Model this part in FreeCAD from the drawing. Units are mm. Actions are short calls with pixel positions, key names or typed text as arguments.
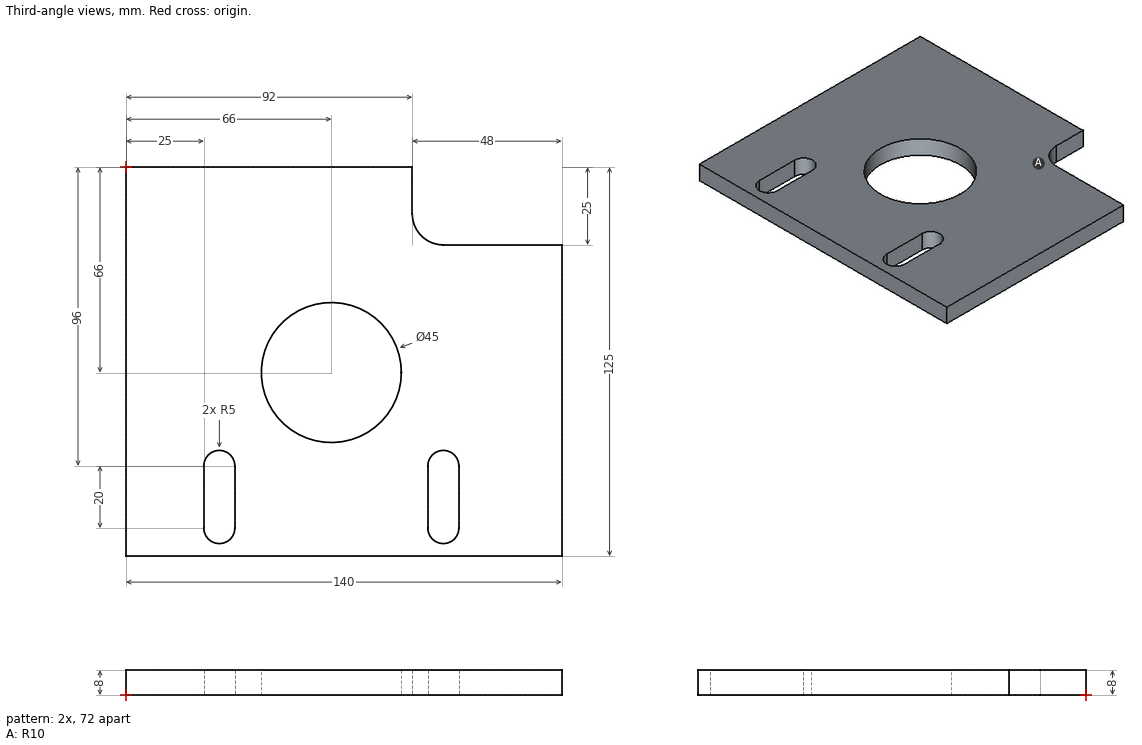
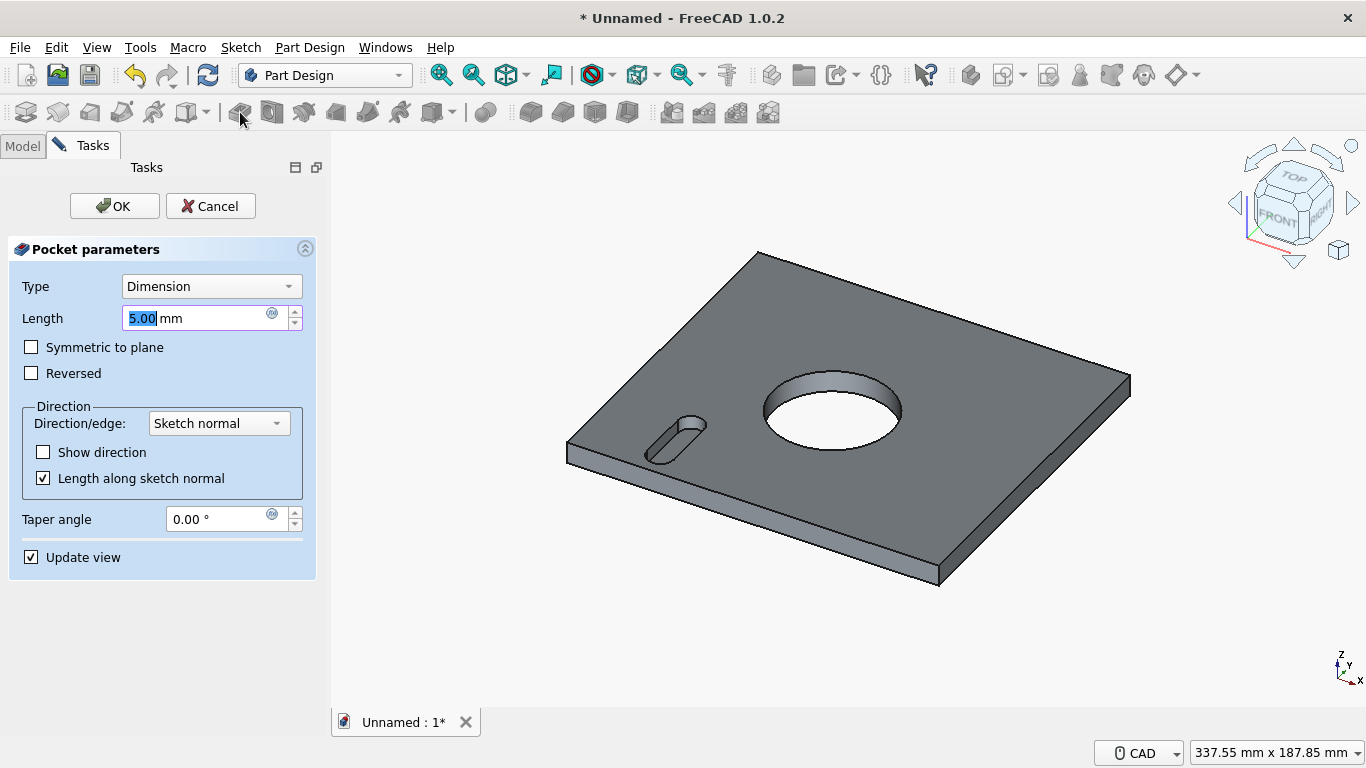
text(8)
key(Tab)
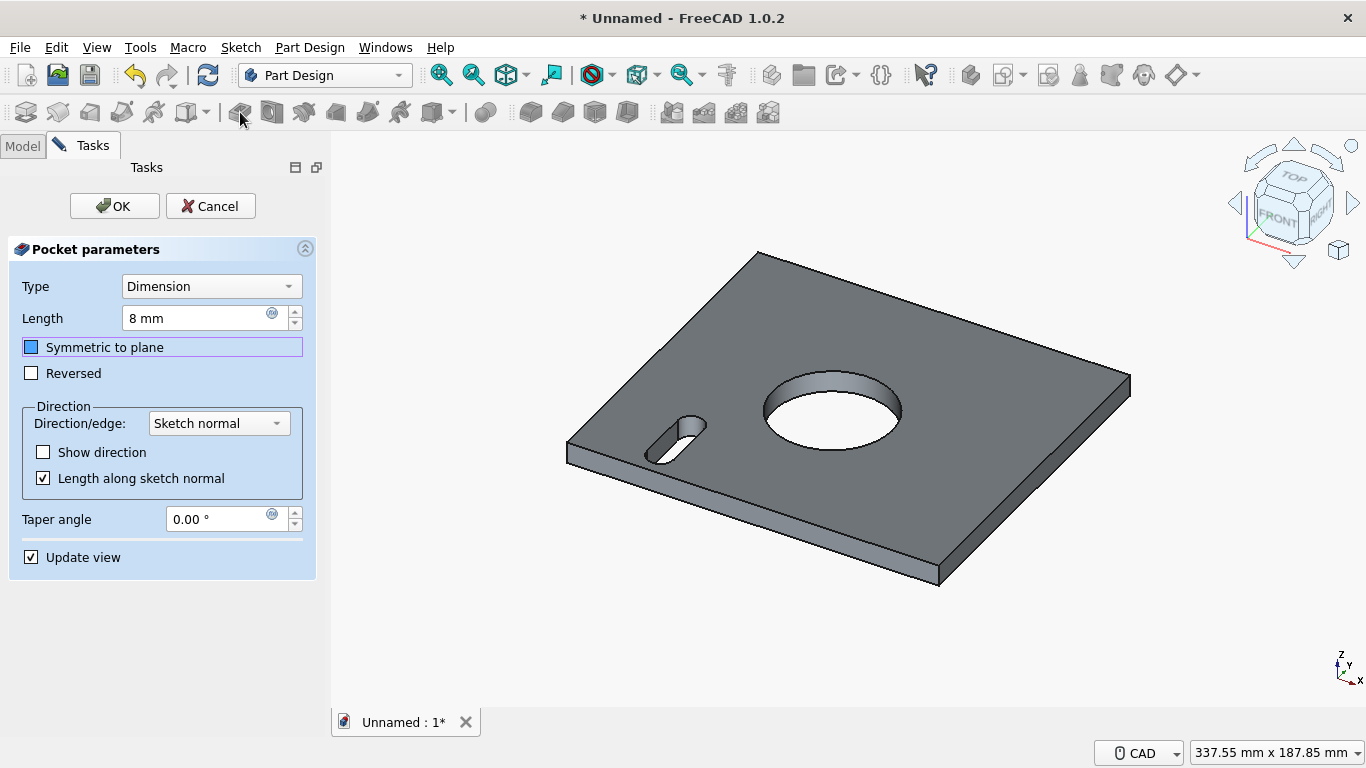
click(115, 206)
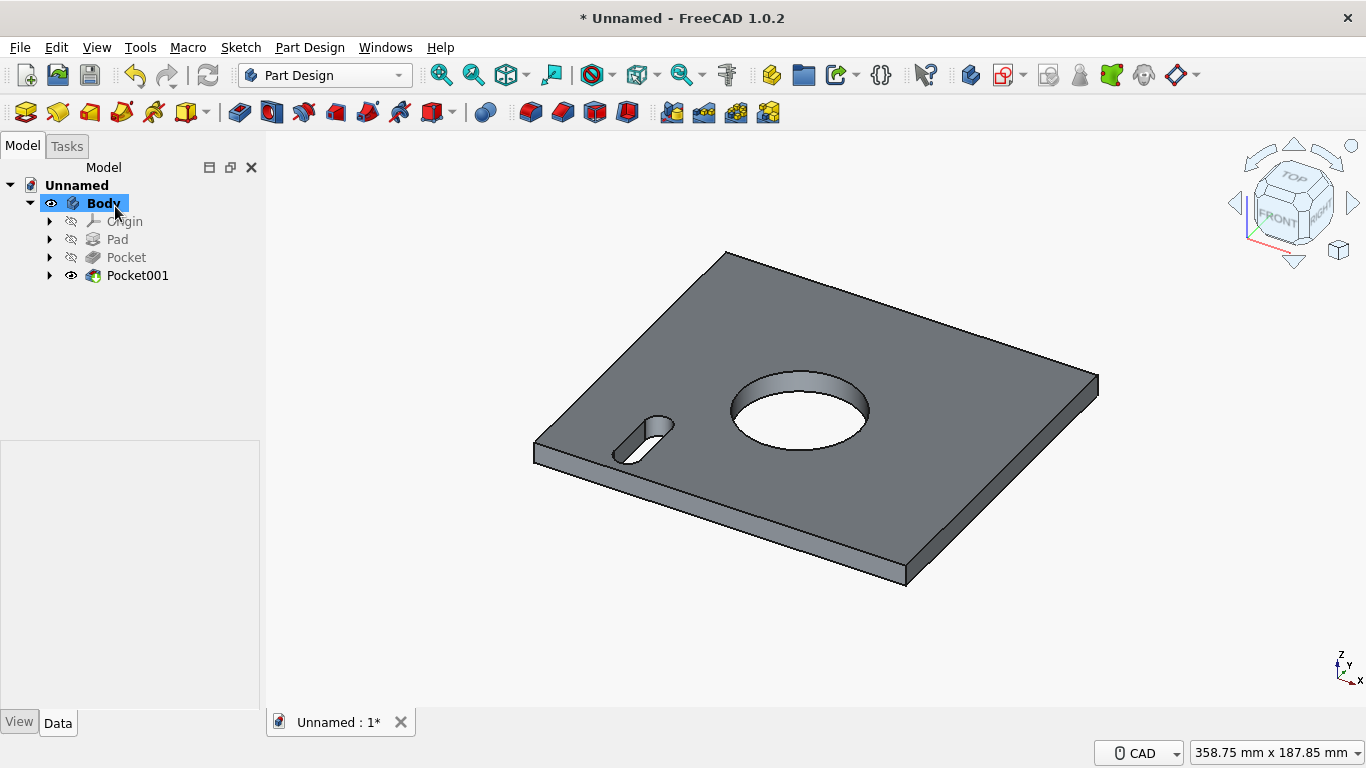
click(116, 275)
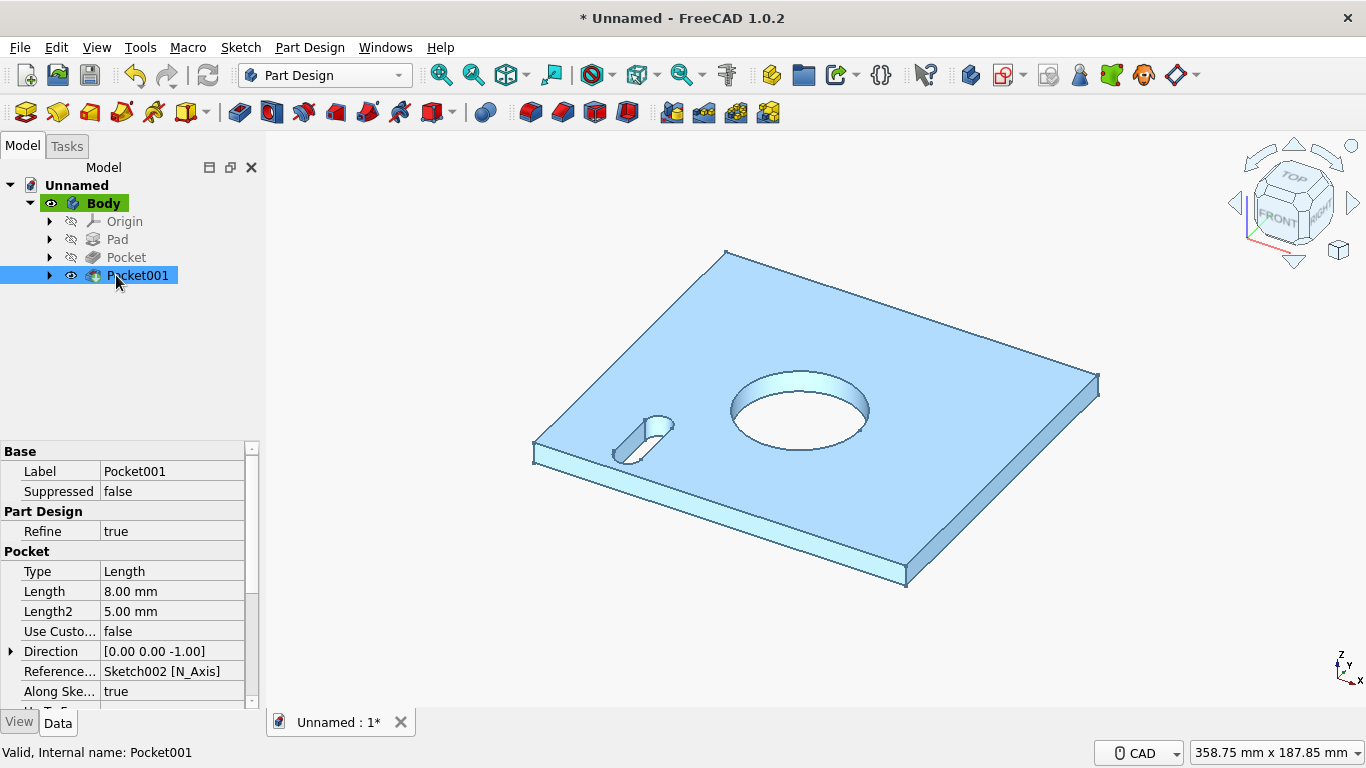
click(704, 112)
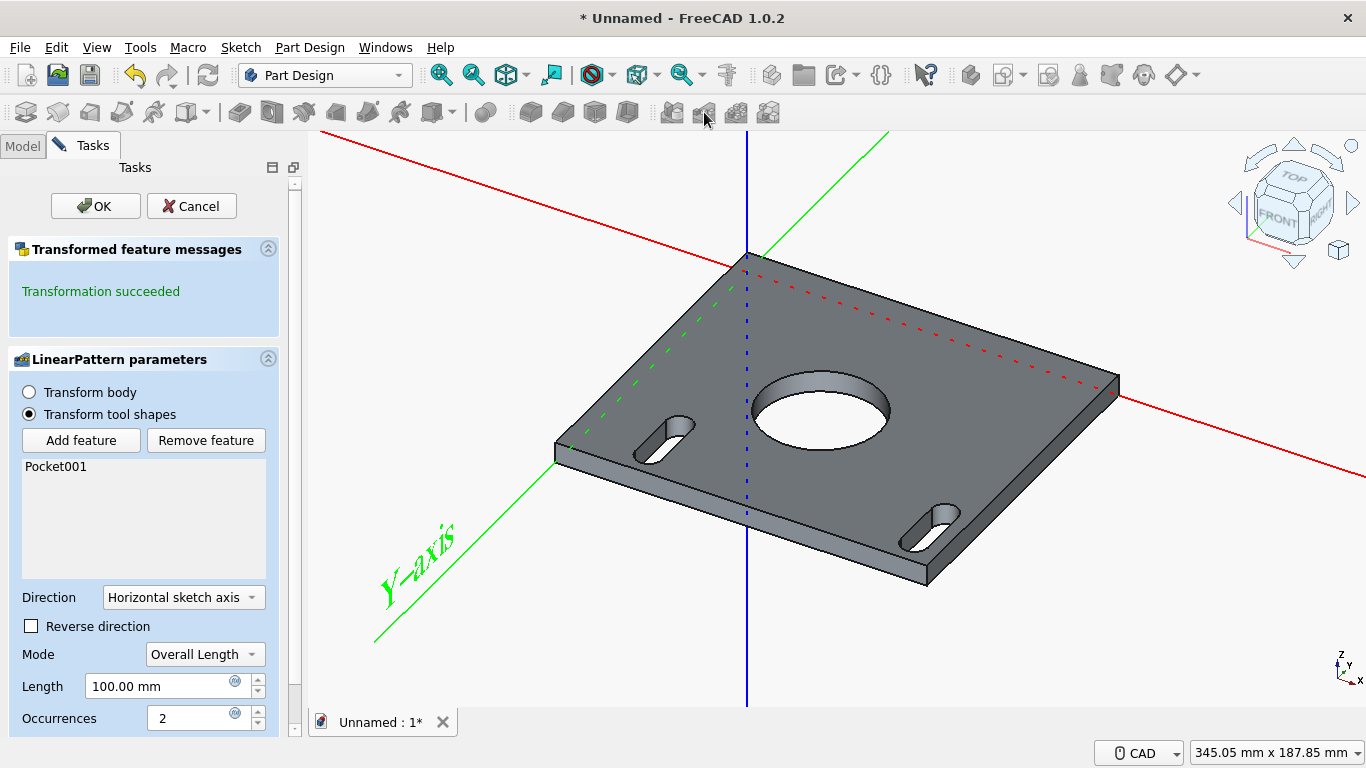
click(184, 598)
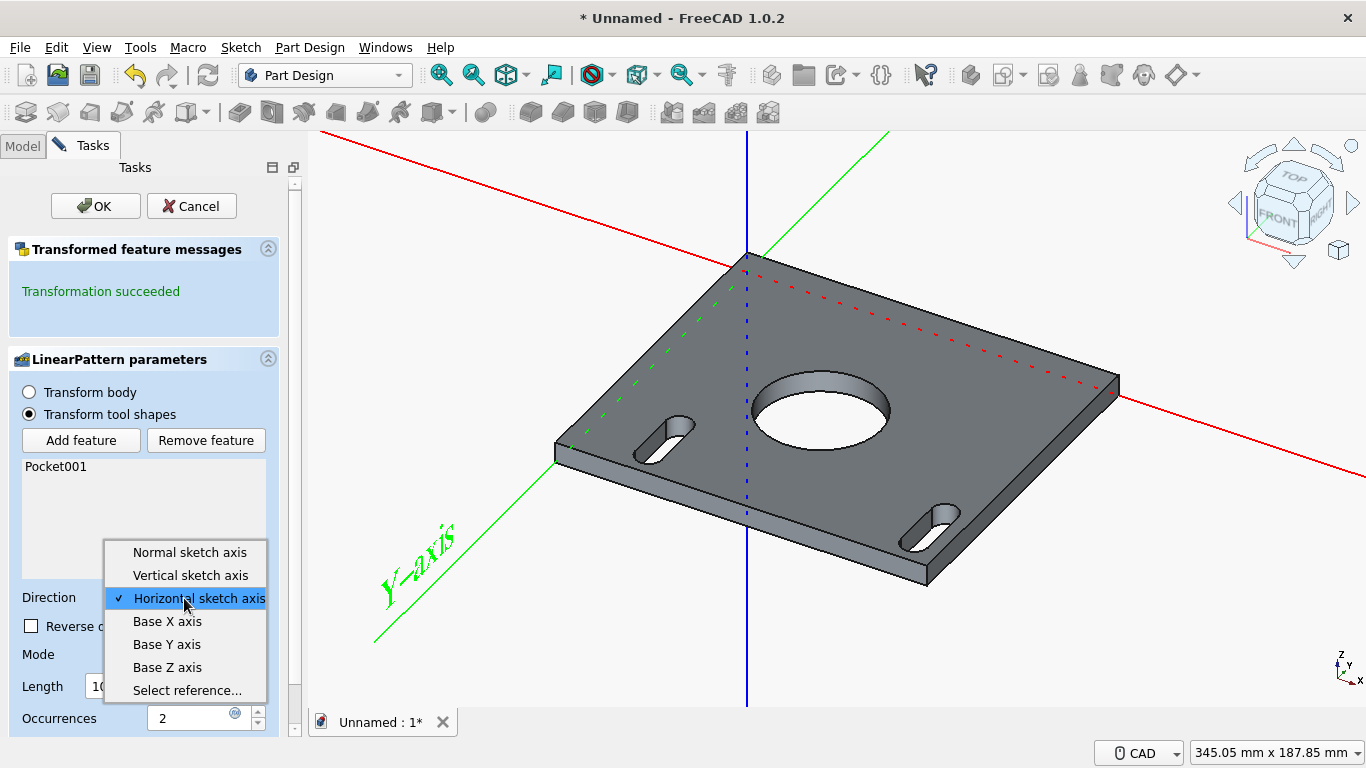
click(184, 622)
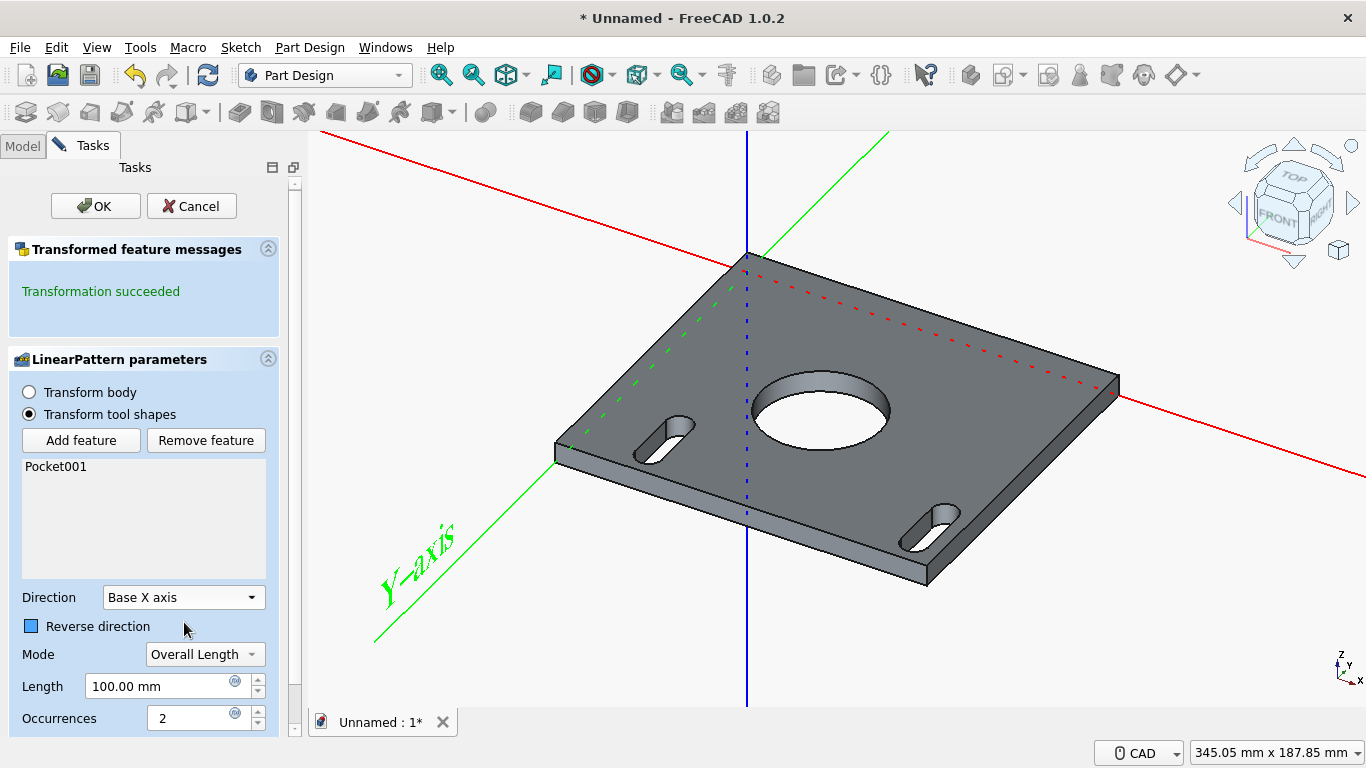
click(206, 654)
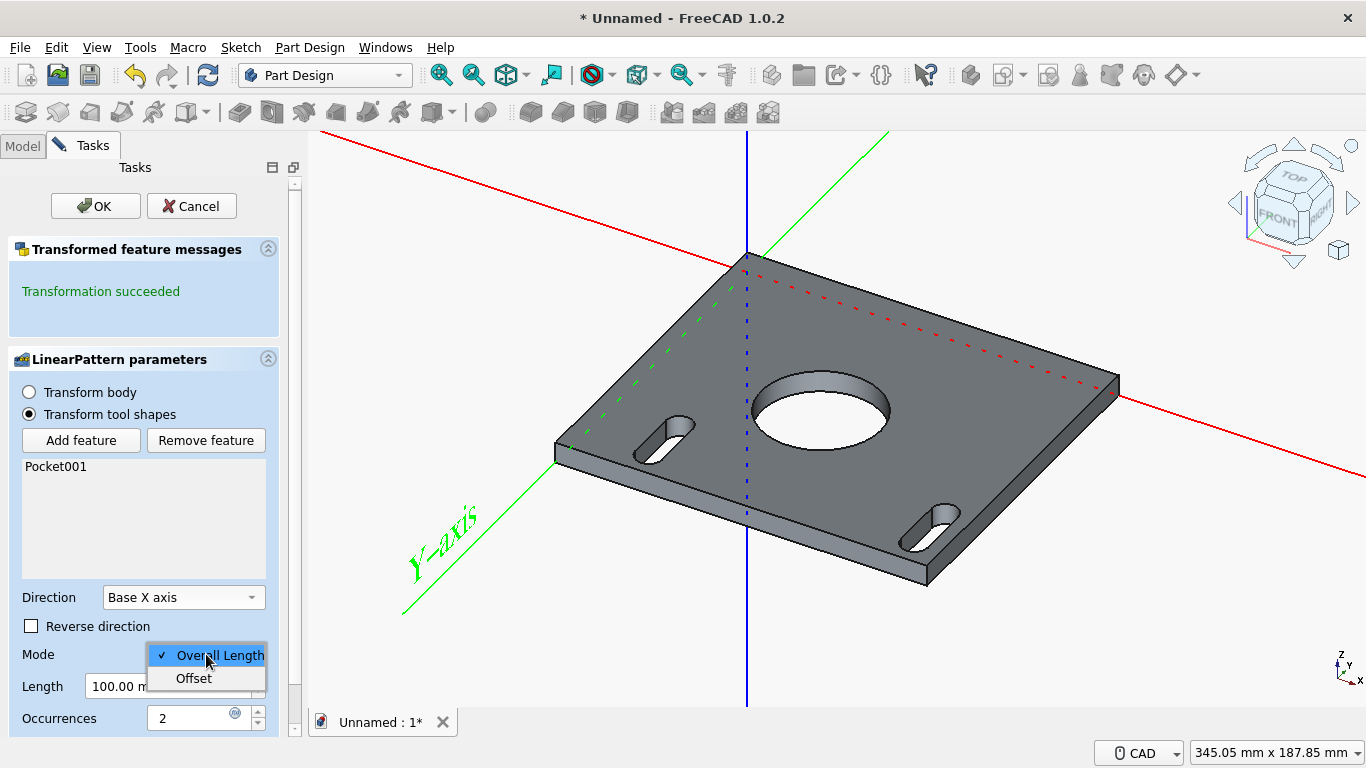
click(206, 678)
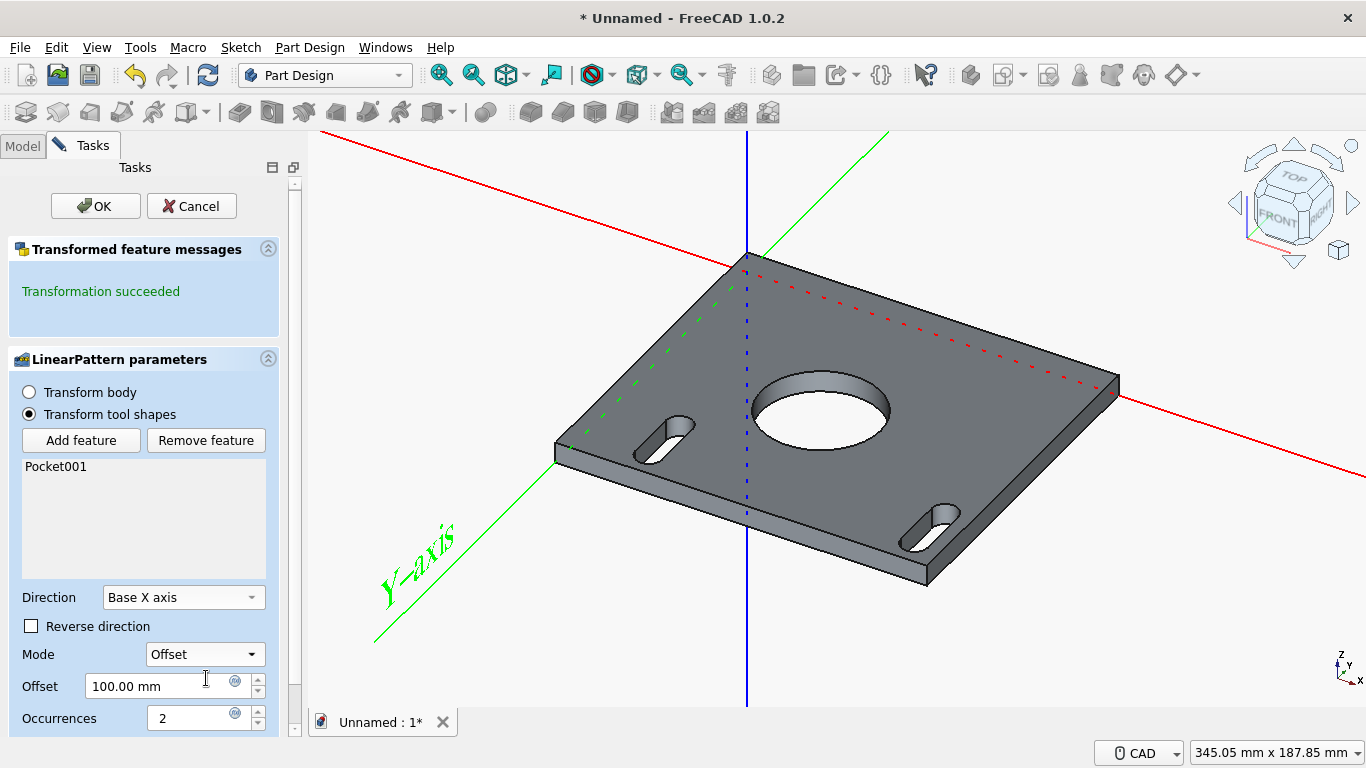
triple_click(168, 686)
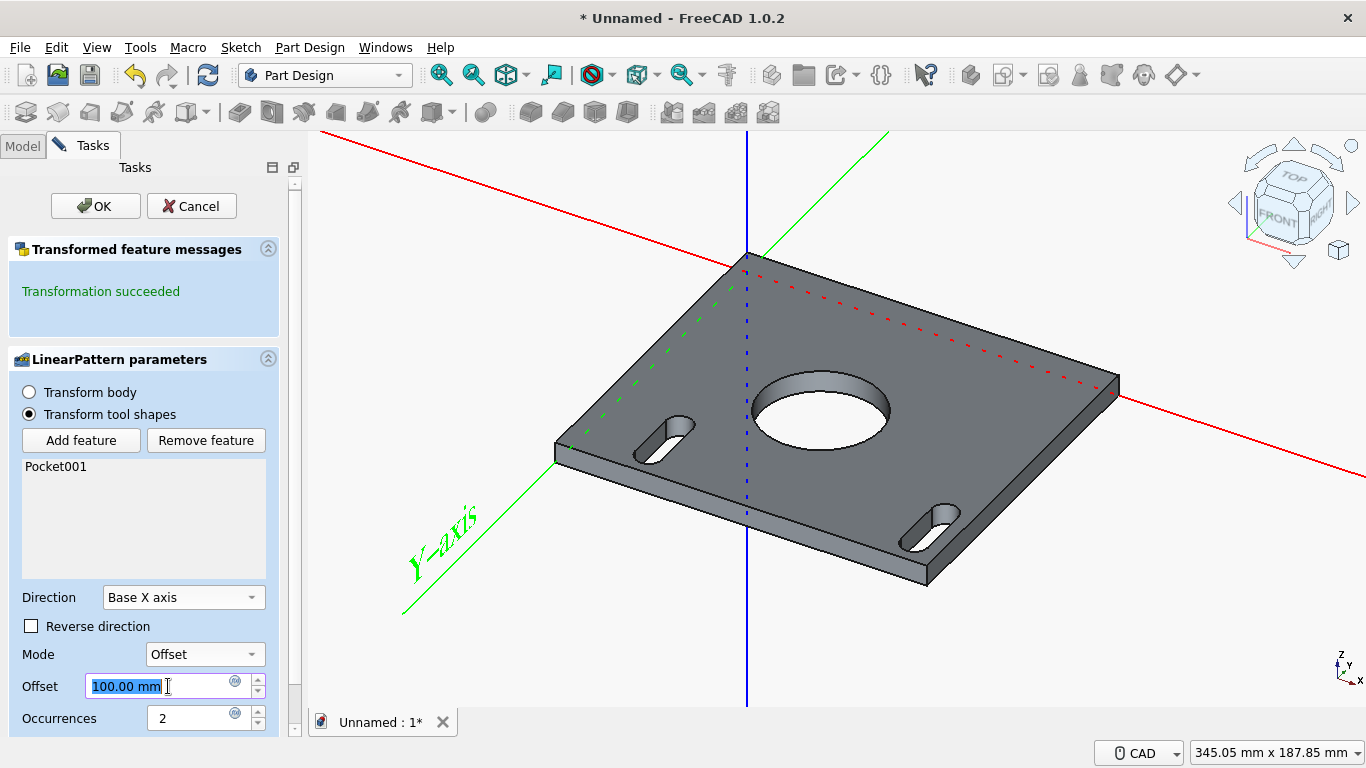
text(72)
key(Tab)